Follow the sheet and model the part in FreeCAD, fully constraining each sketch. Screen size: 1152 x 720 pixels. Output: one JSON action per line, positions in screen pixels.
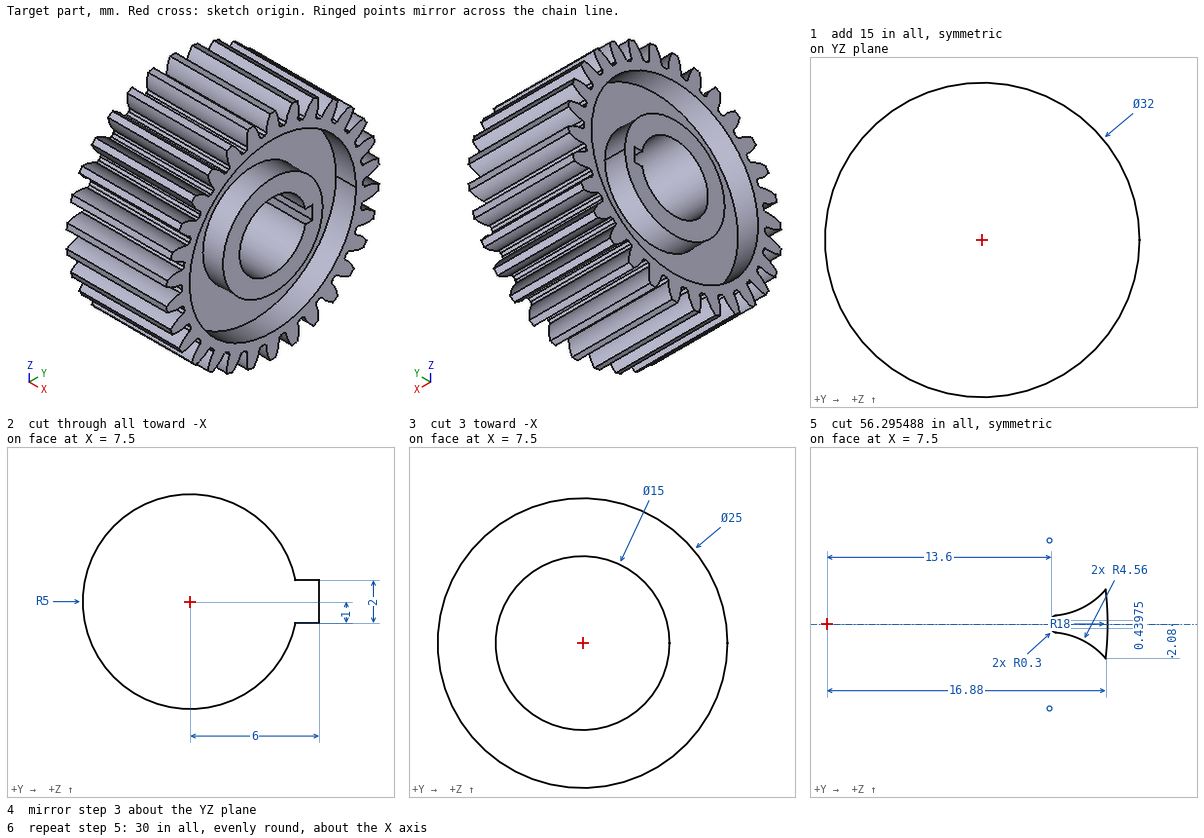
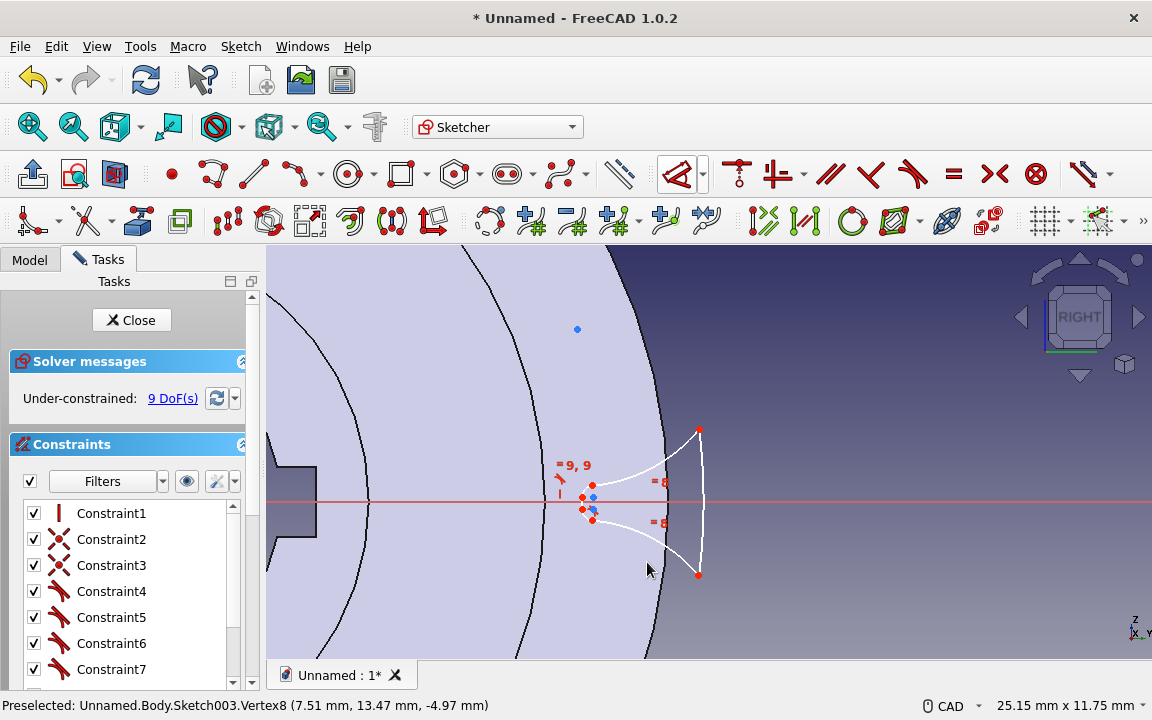
{"action": "left_click", "coordinate": [578, 329]}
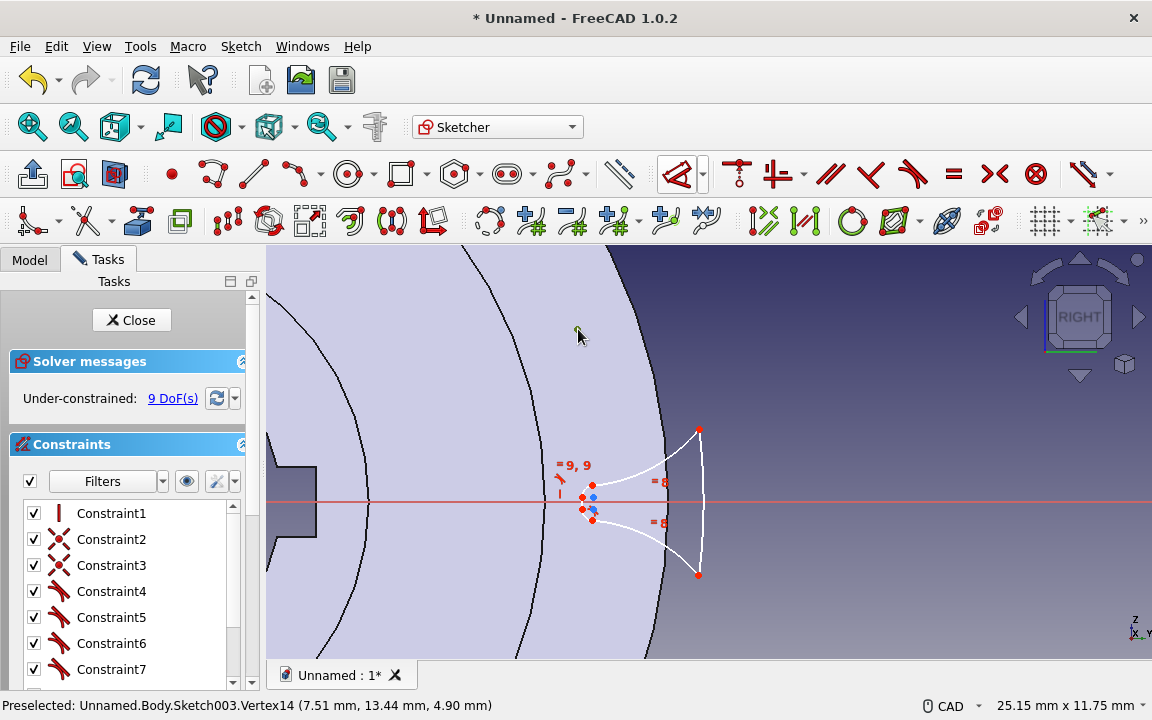
{"action": "left_click", "coordinate": [344, 502]}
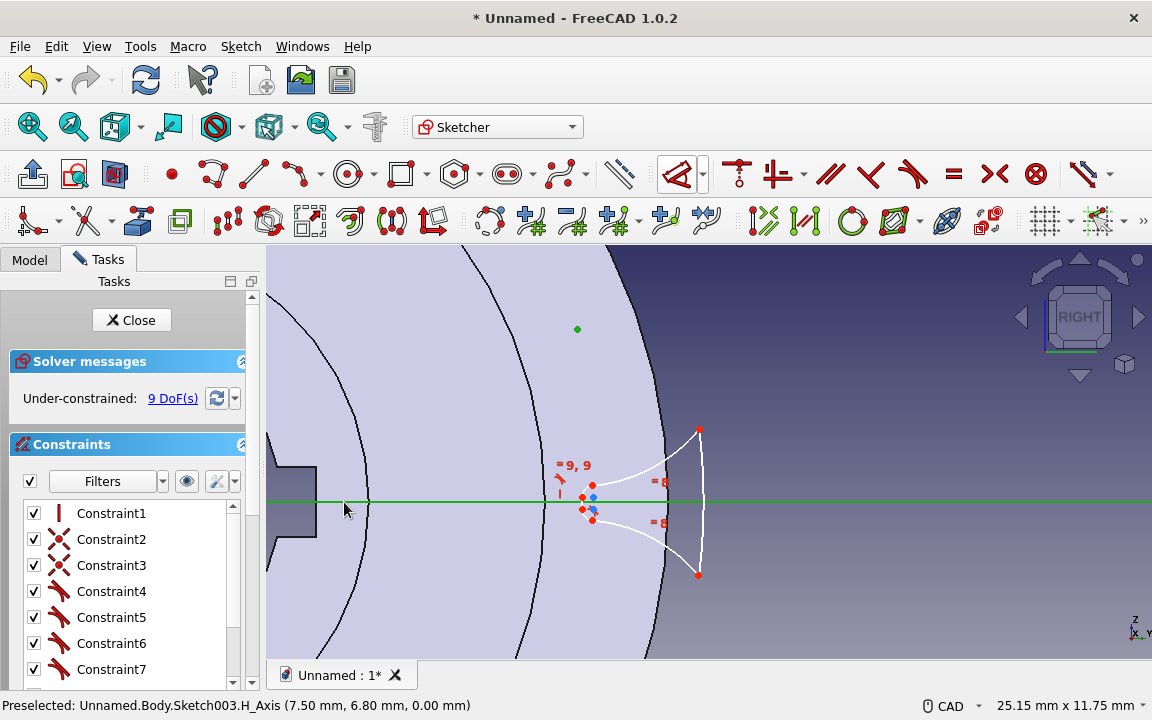
{"action": "left_click", "coordinate": [995, 174]}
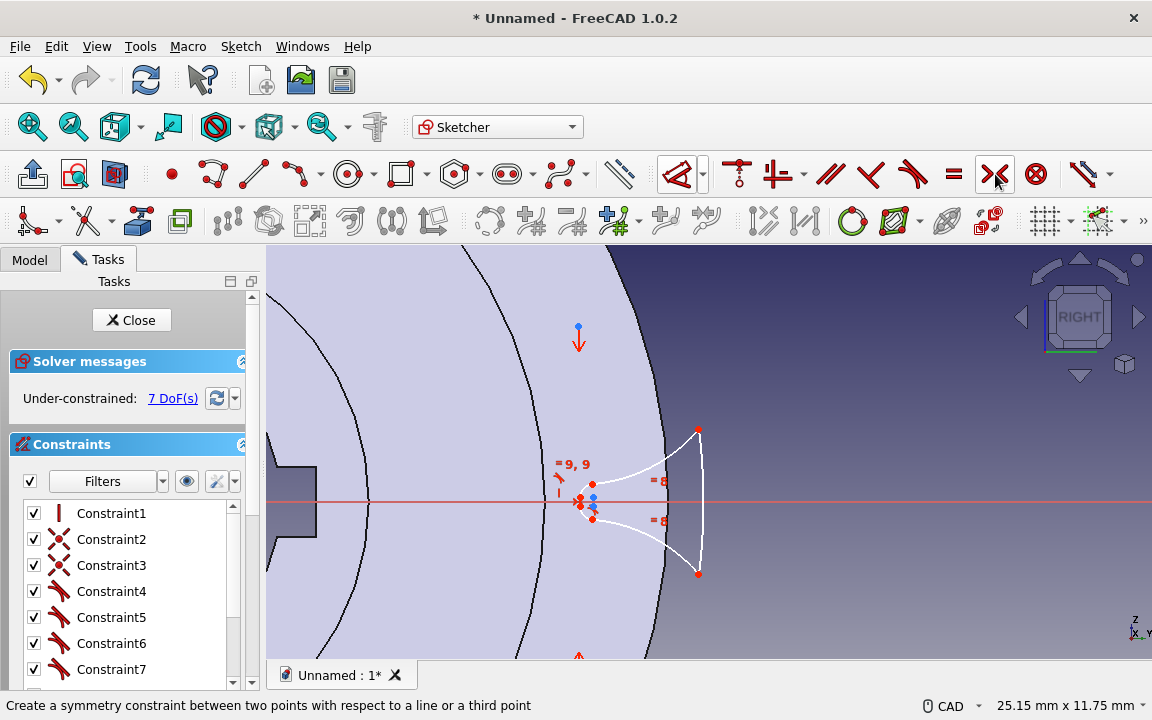
{"action": "scroll", "coordinate": [584, 516], "scroll_direction": "up", "scroll_amount": 7}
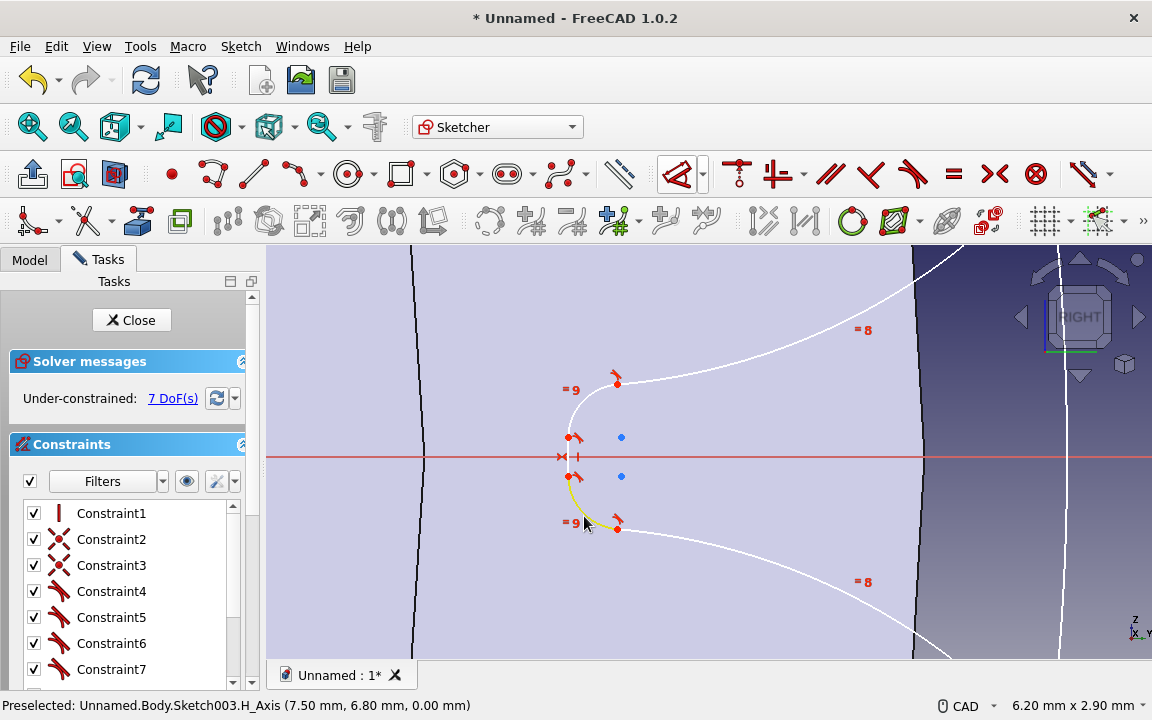
{"action": "left_click", "coordinate": [583, 512]}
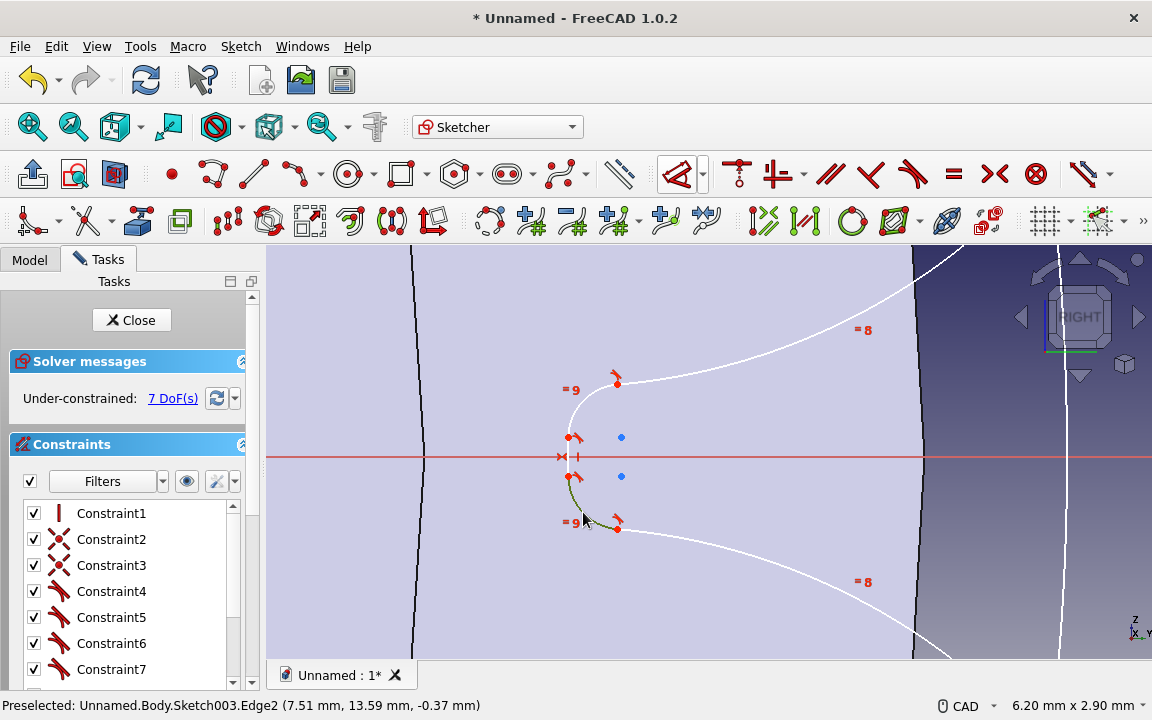
{"action": "key", "text": "k r"}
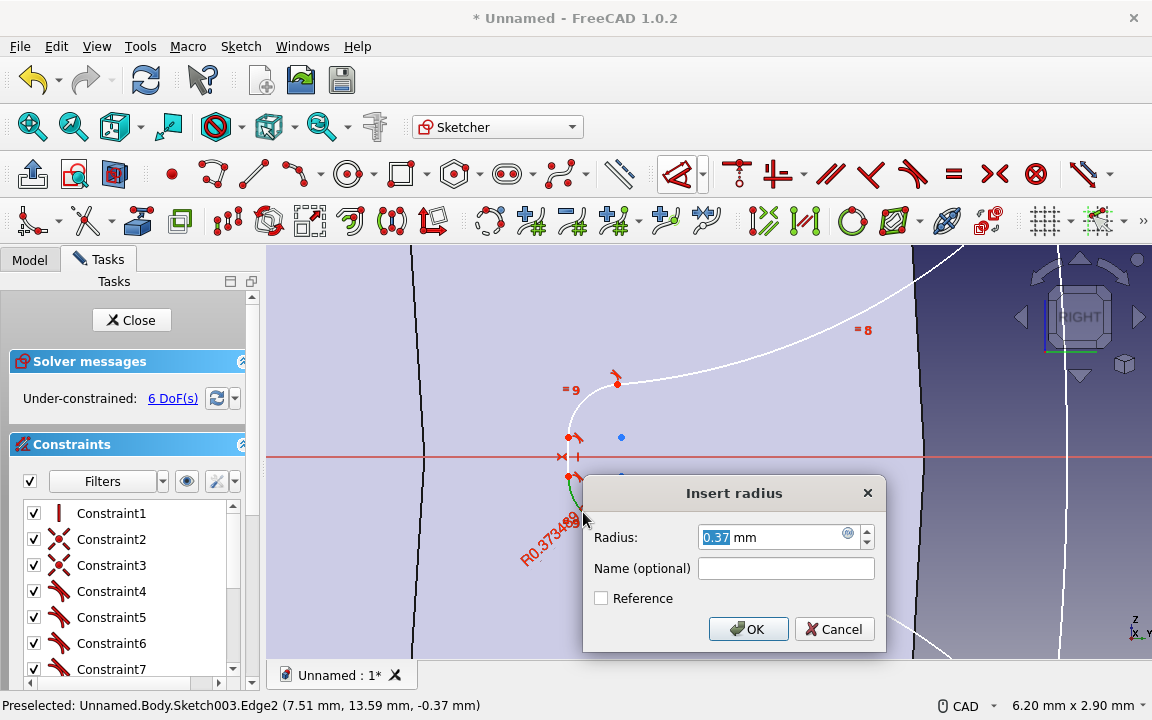
{"action": "type", "text": "0.3"}
{"action": "key", "text": "Return"}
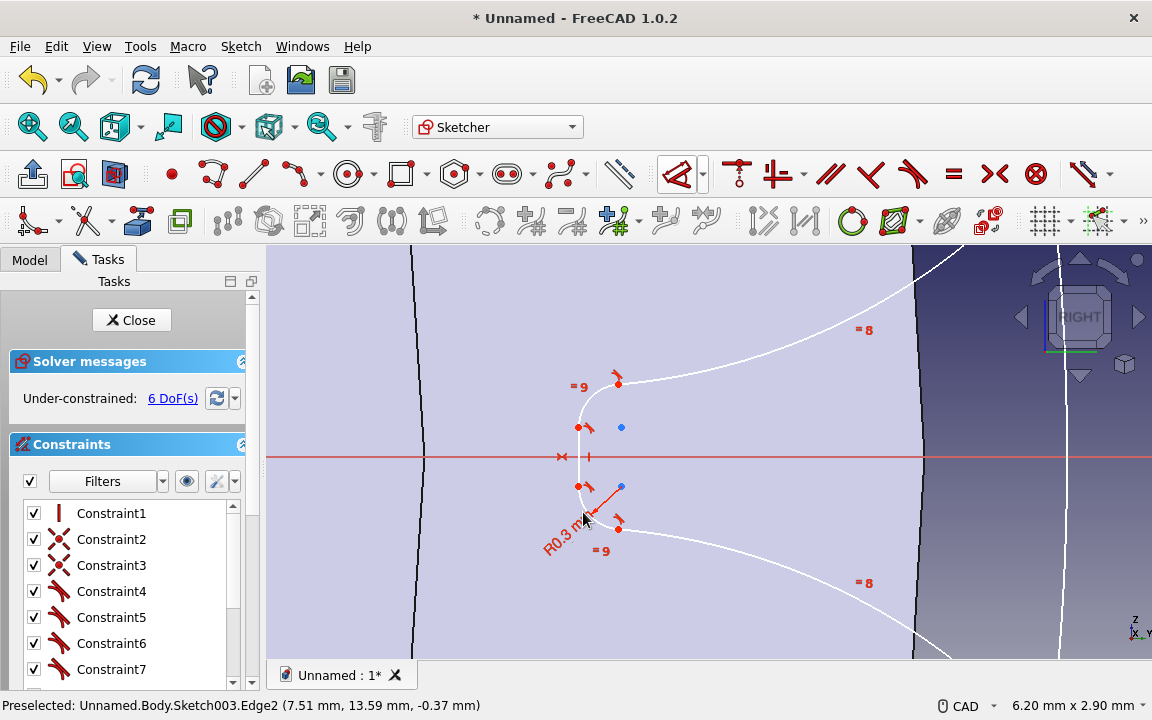
{"action": "left_click", "coordinate": [764, 559]}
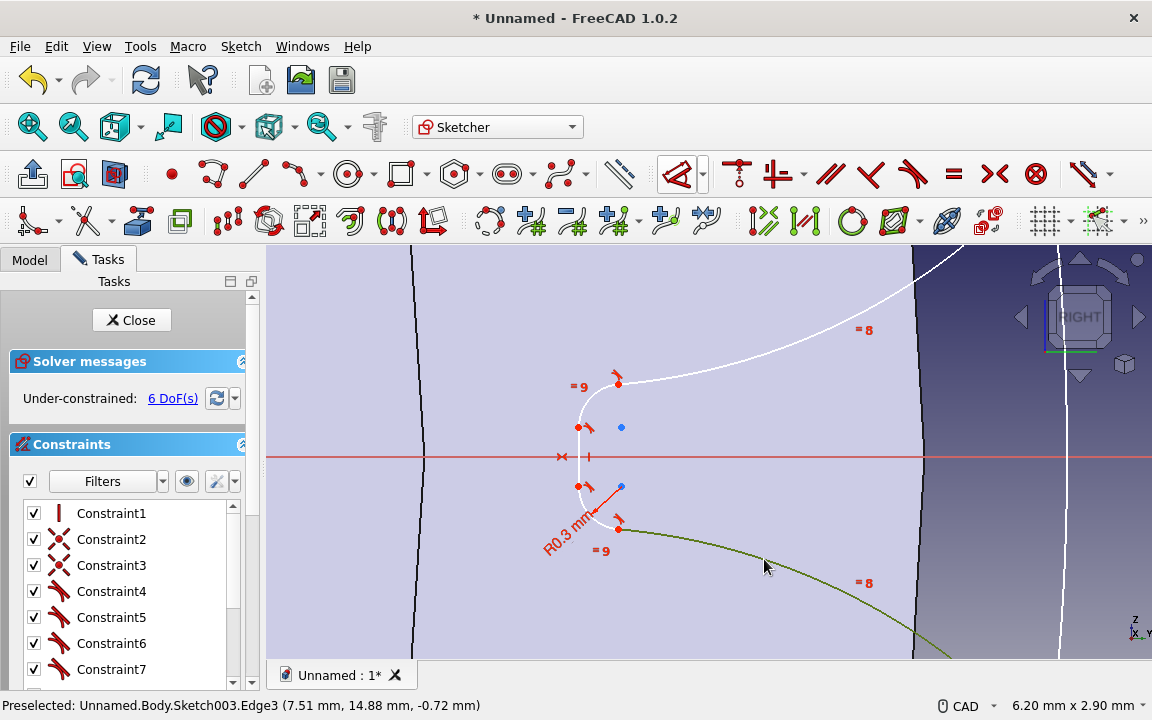
{"action": "left_click", "coordinate": [702, 174]}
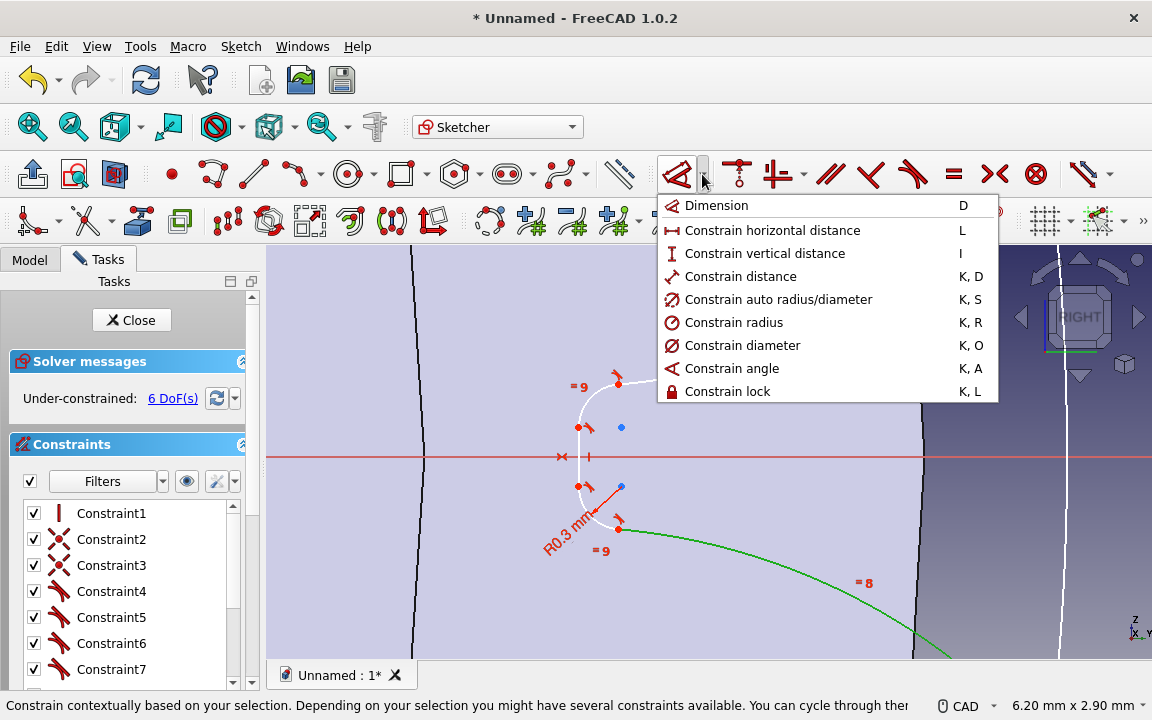
{"action": "left_click", "coordinate": [828, 322]}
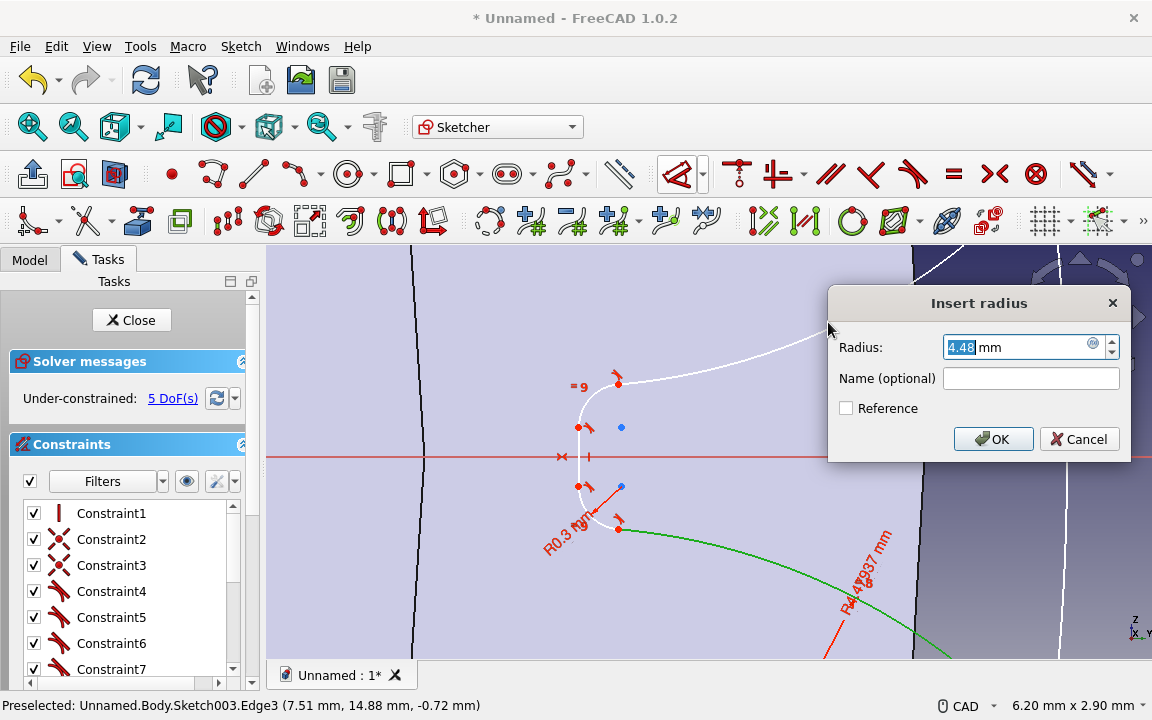
{"action": "type", "text": "4.56"}
{"action": "key", "text": "Return"}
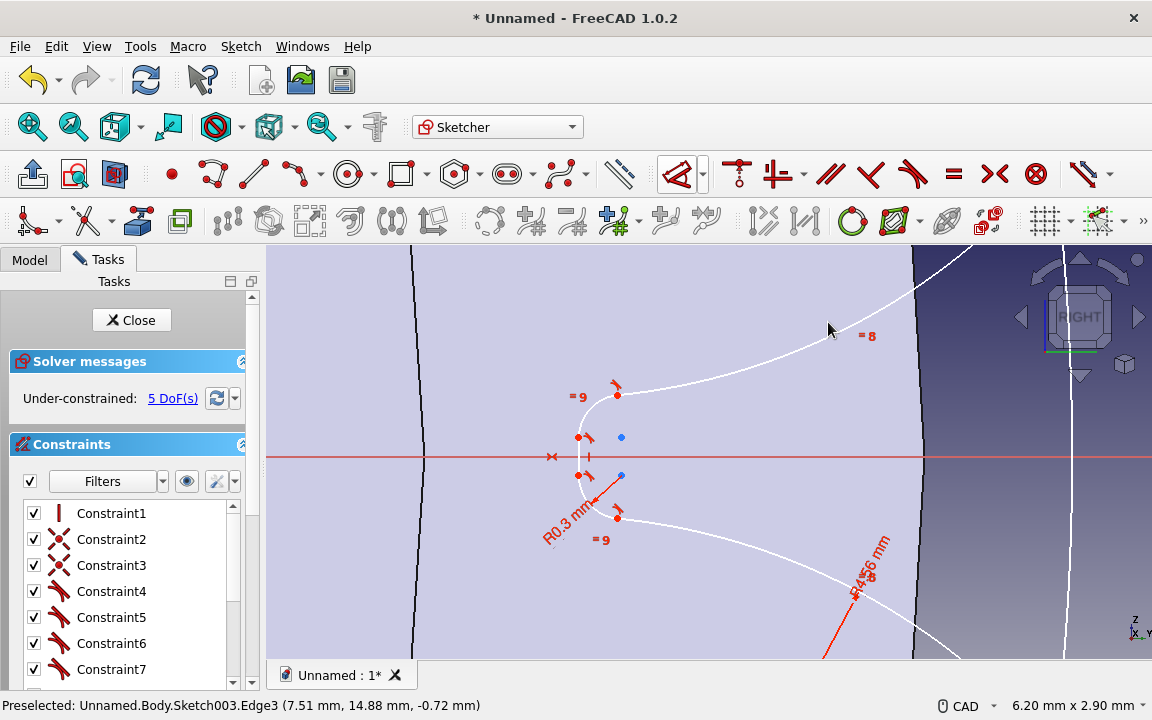
{"action": "scroll", "coordinate": [490, 448], "scroll_direction": "down", "scroll_amount": 4}